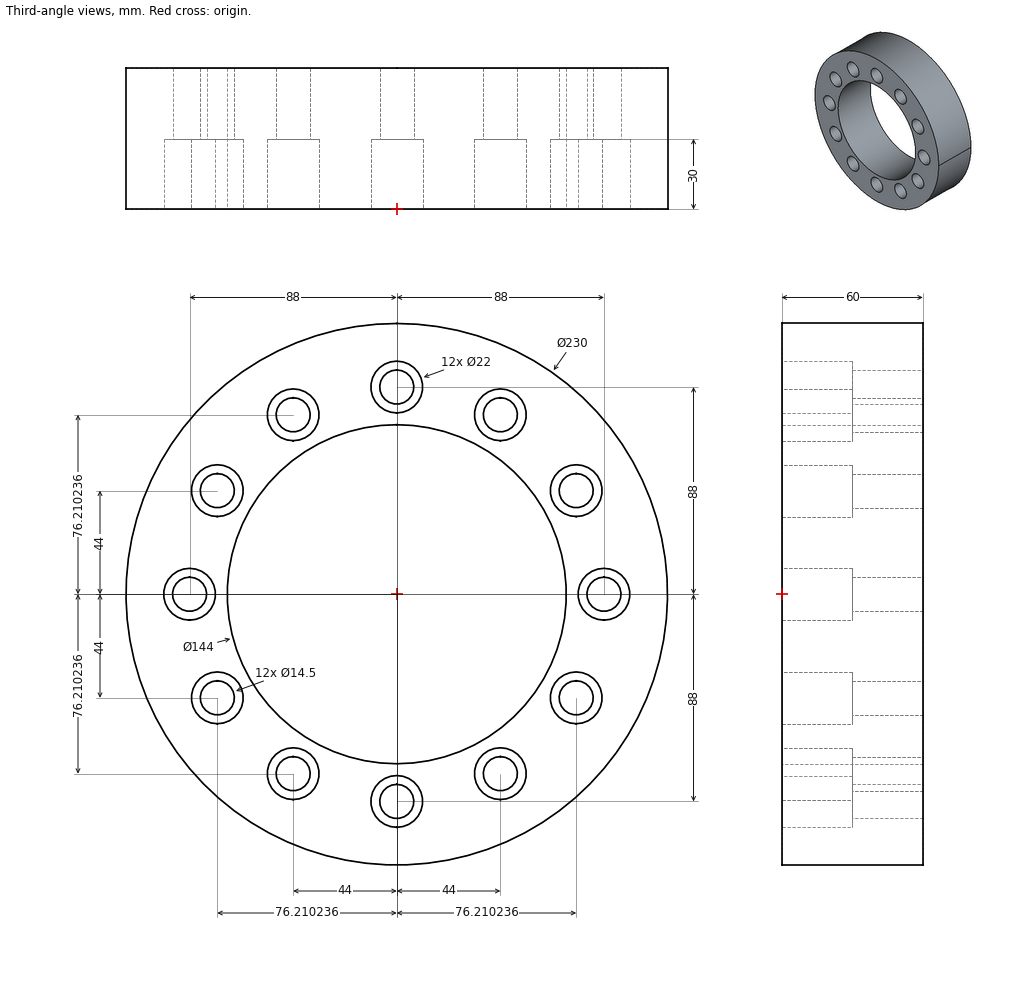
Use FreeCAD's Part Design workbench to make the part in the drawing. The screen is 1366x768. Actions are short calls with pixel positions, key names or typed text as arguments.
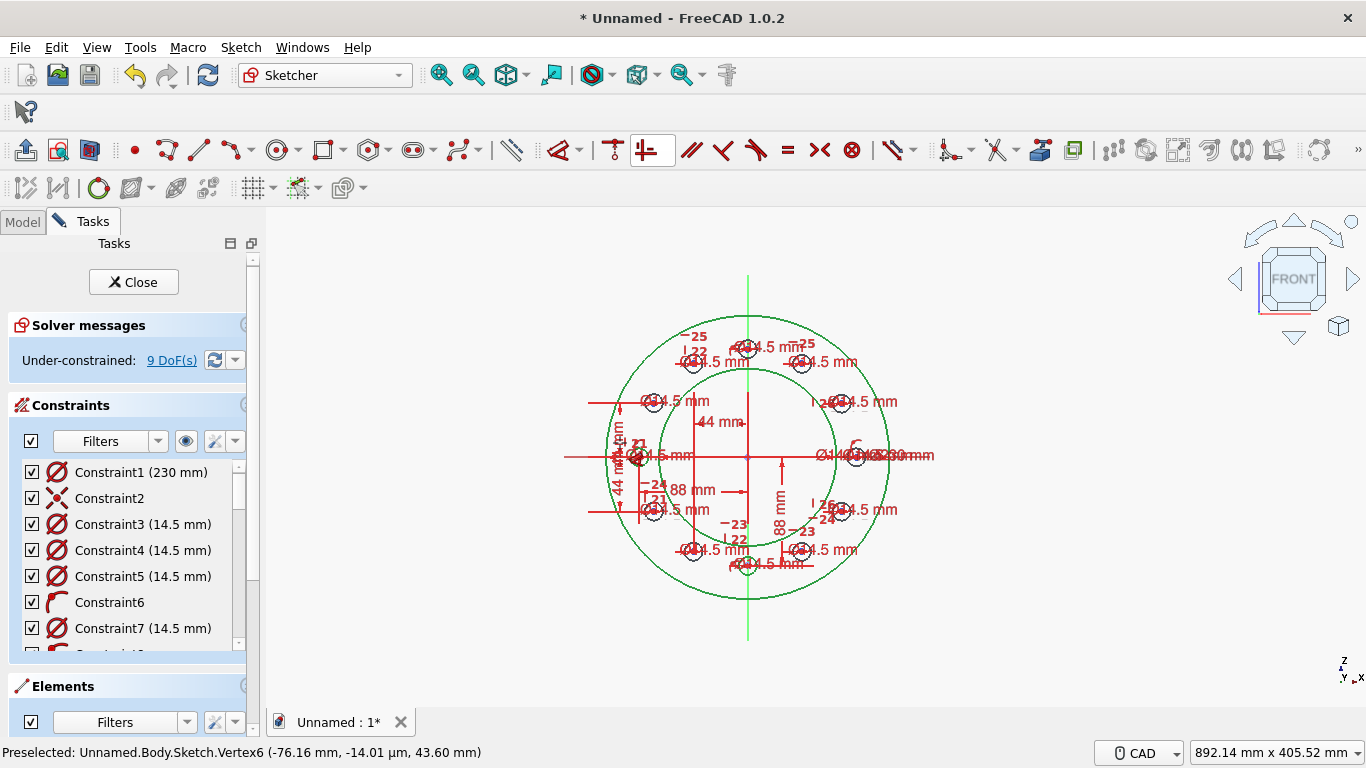
click(802, 552)
click(794, 423)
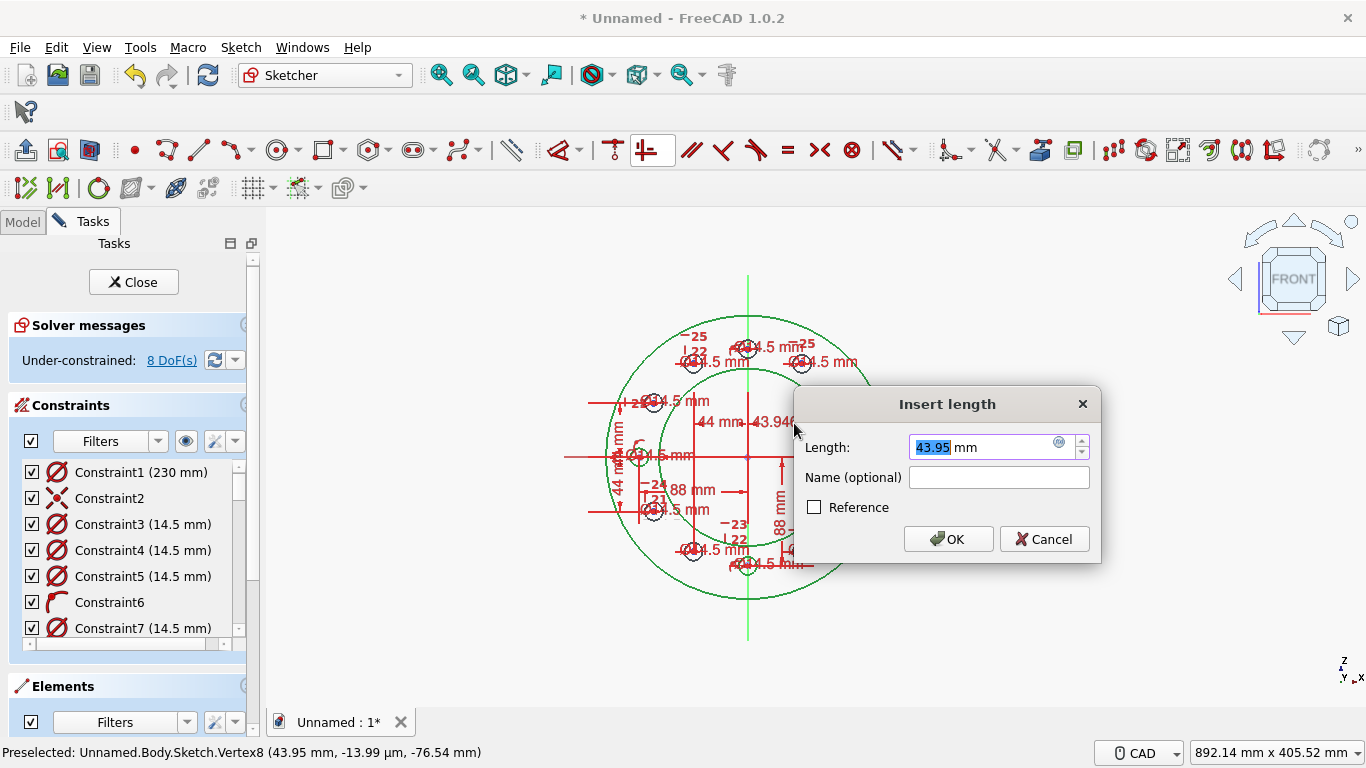
text(44)
key(Return)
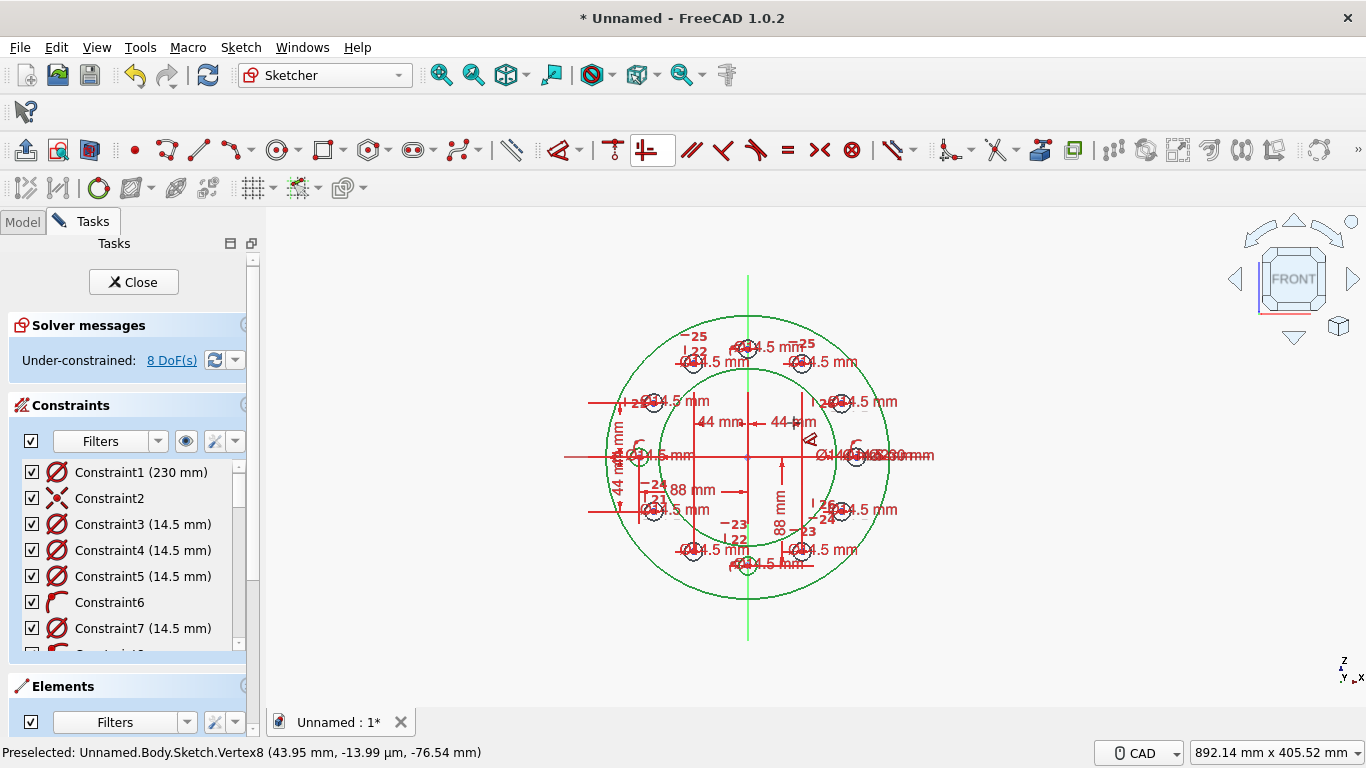
click(856, 457)
click(802, 491)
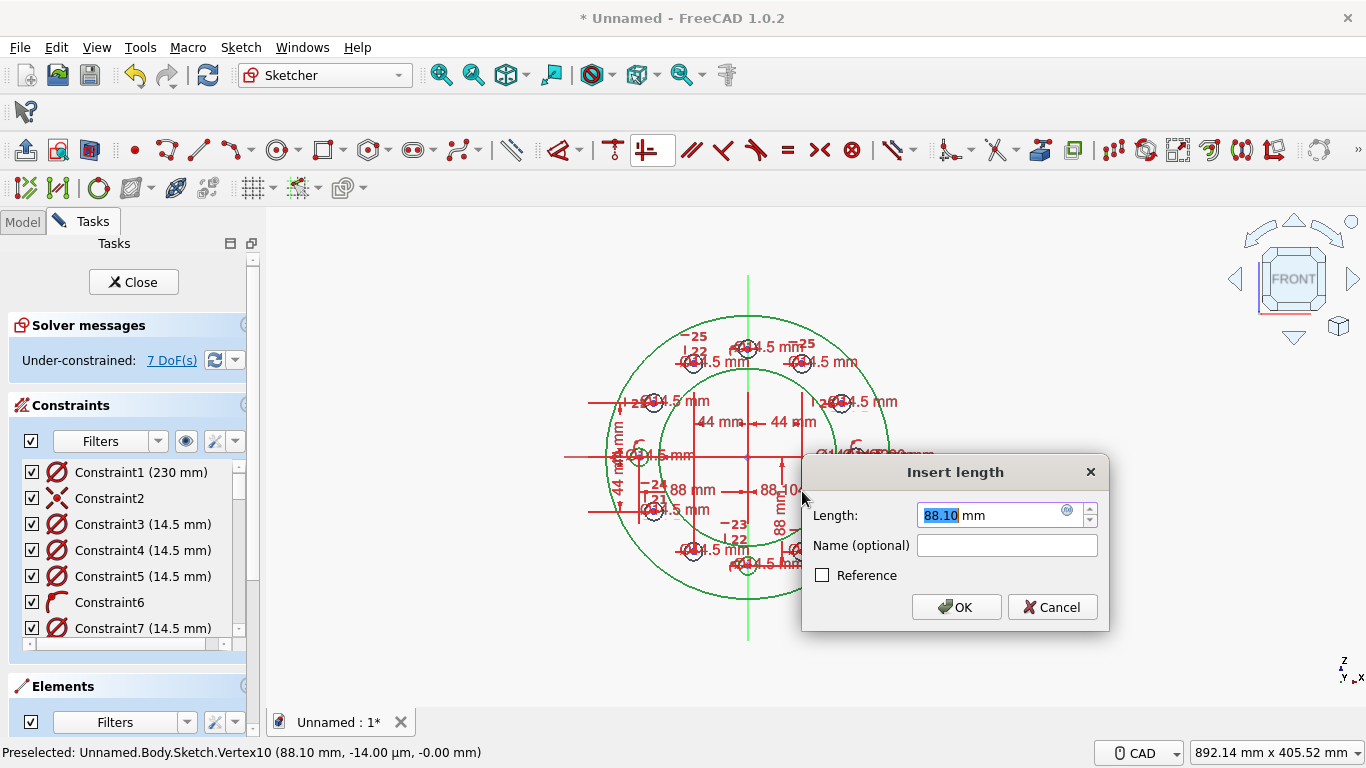
text(88)
key(Return)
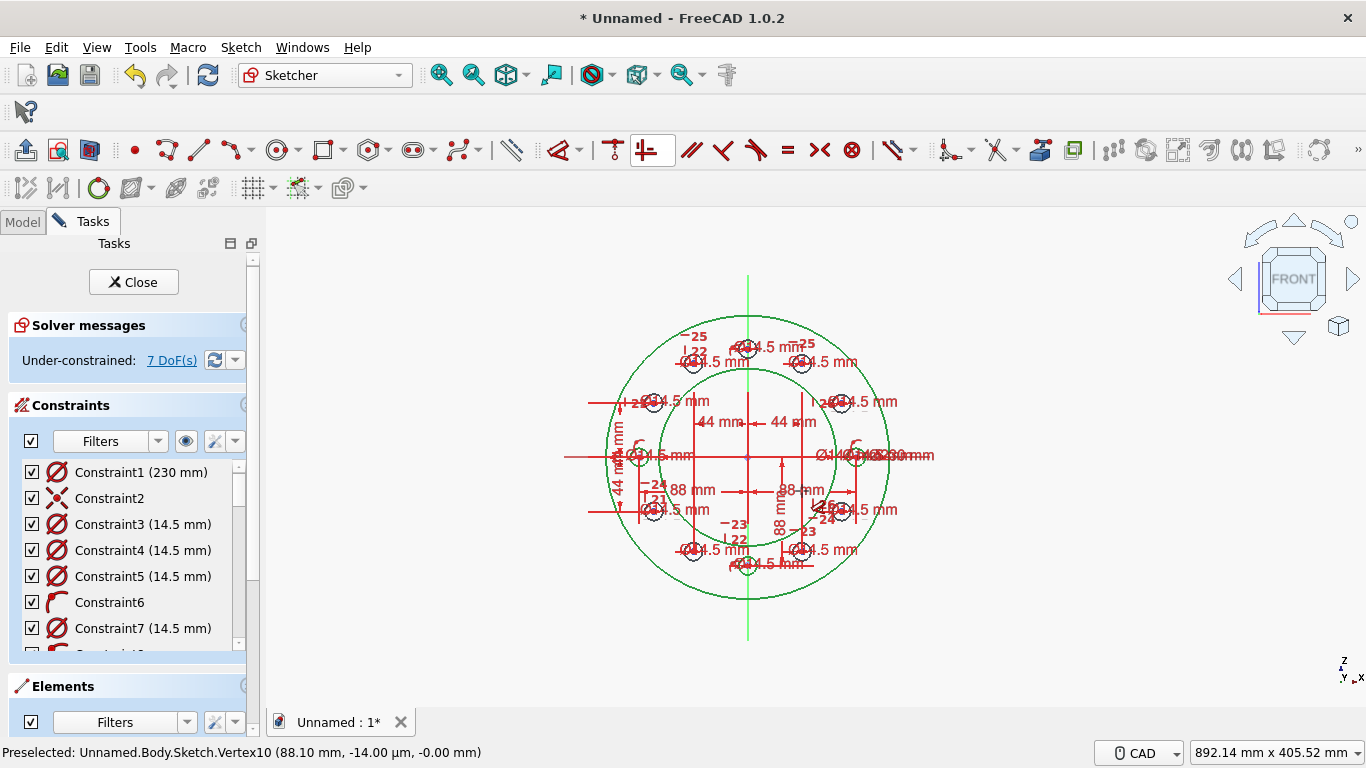
click(748, 349)
click(782, 403)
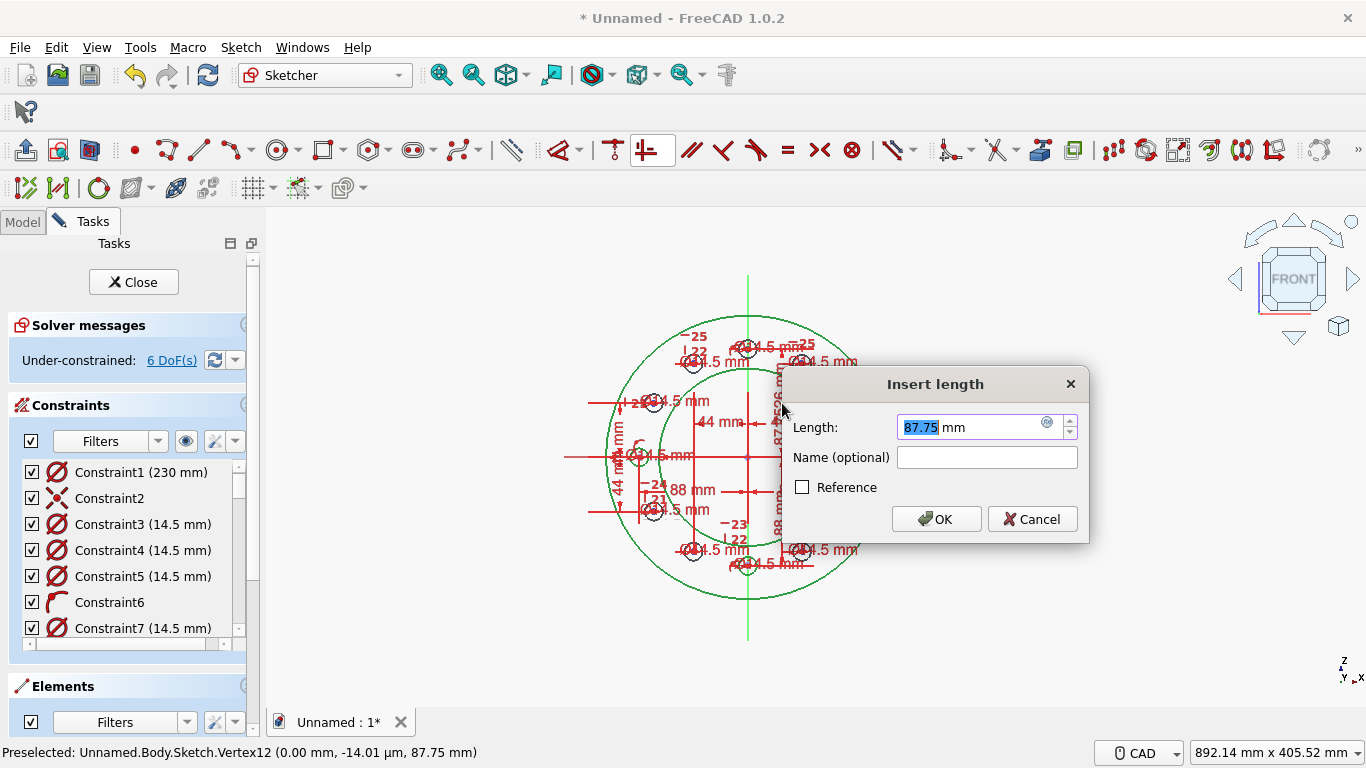
text(88)
key(Return)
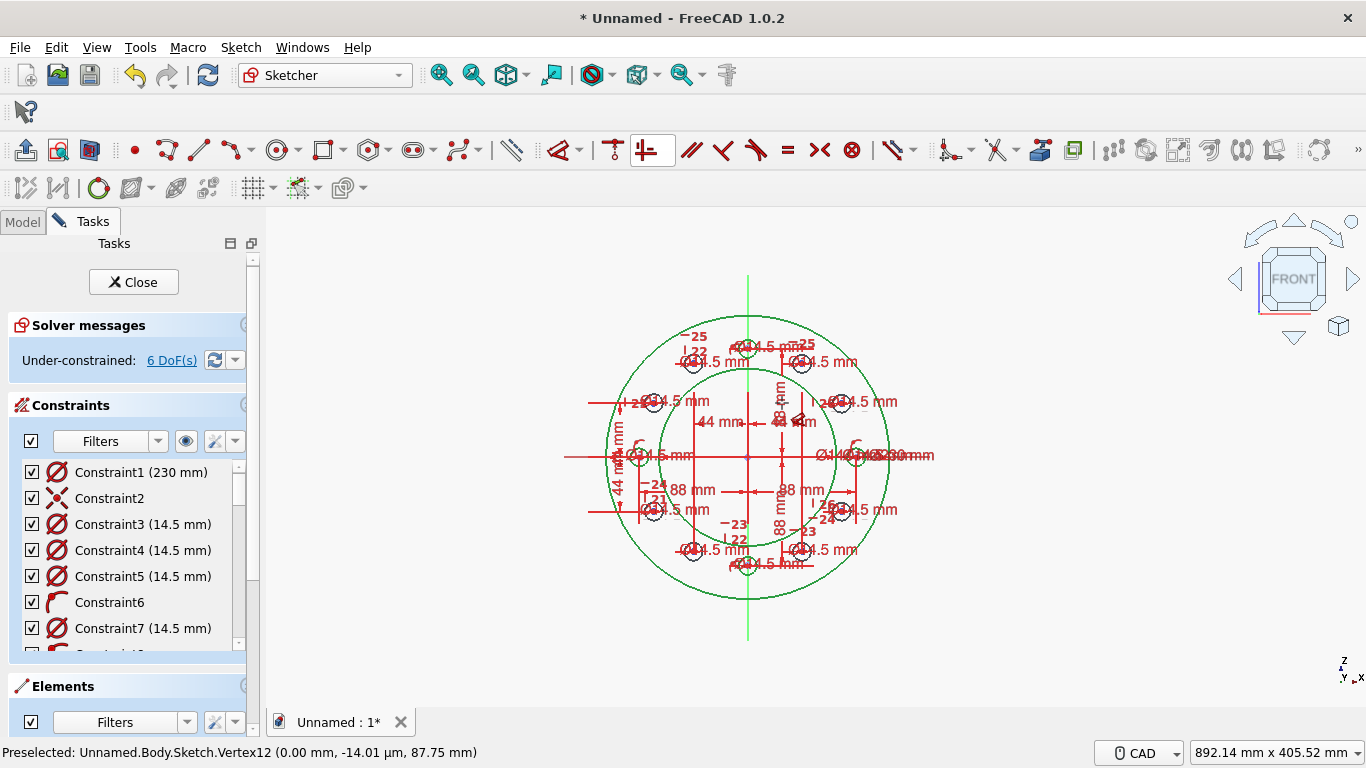
click(802, 364)
click(762, 330)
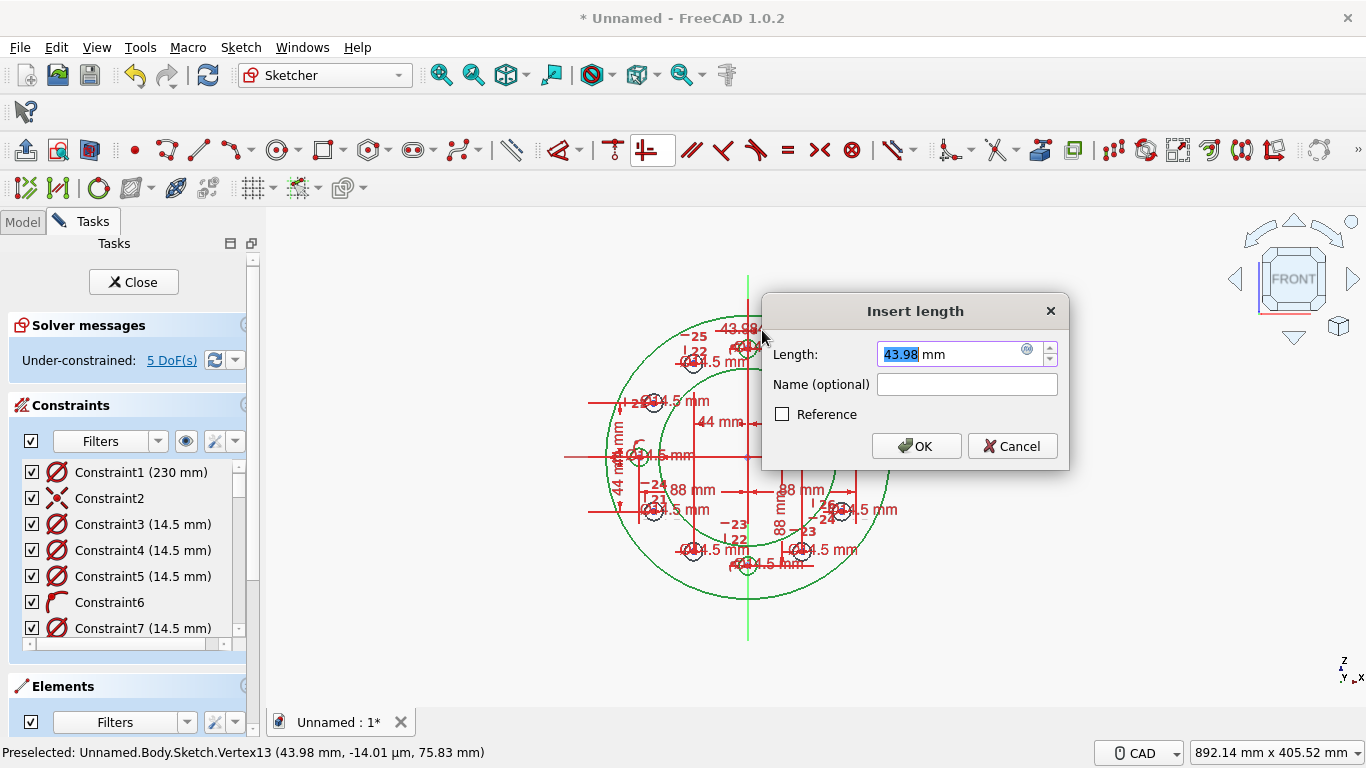
text(44)
key(Return)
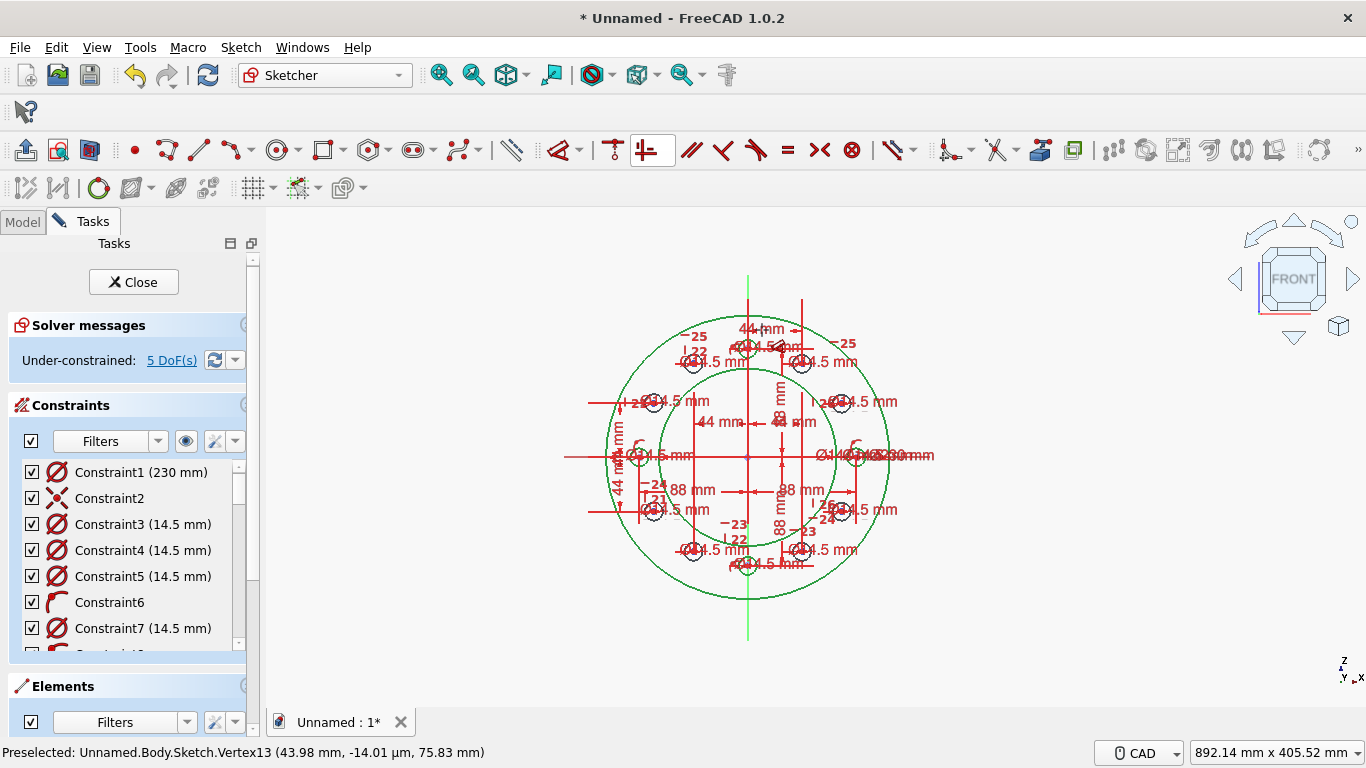
click(842, 404)
click(876, 443)